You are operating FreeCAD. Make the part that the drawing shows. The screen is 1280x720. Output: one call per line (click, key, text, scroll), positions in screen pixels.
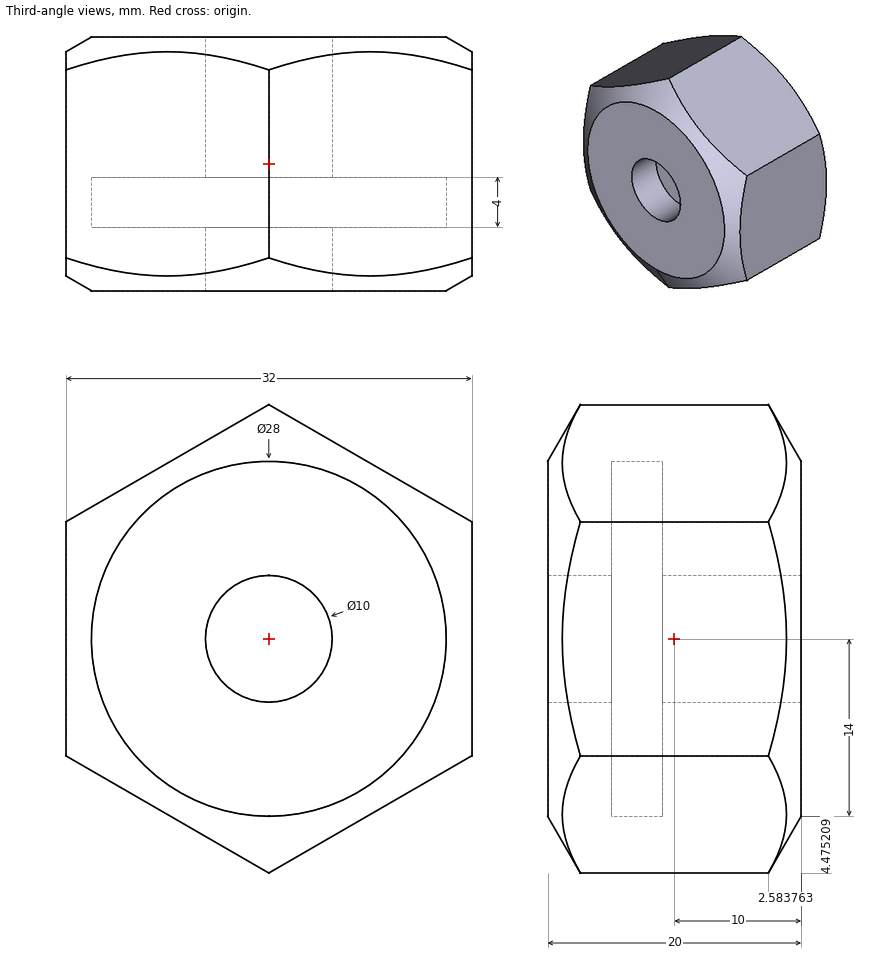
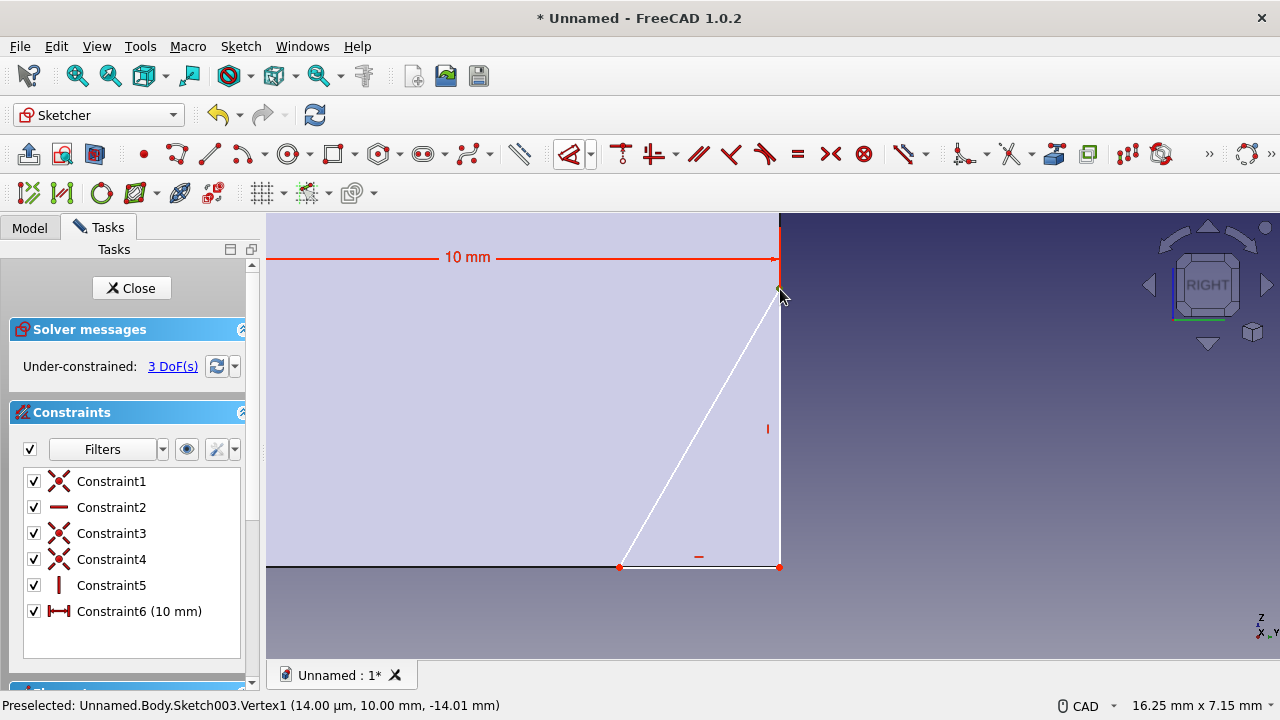
click(590, 154)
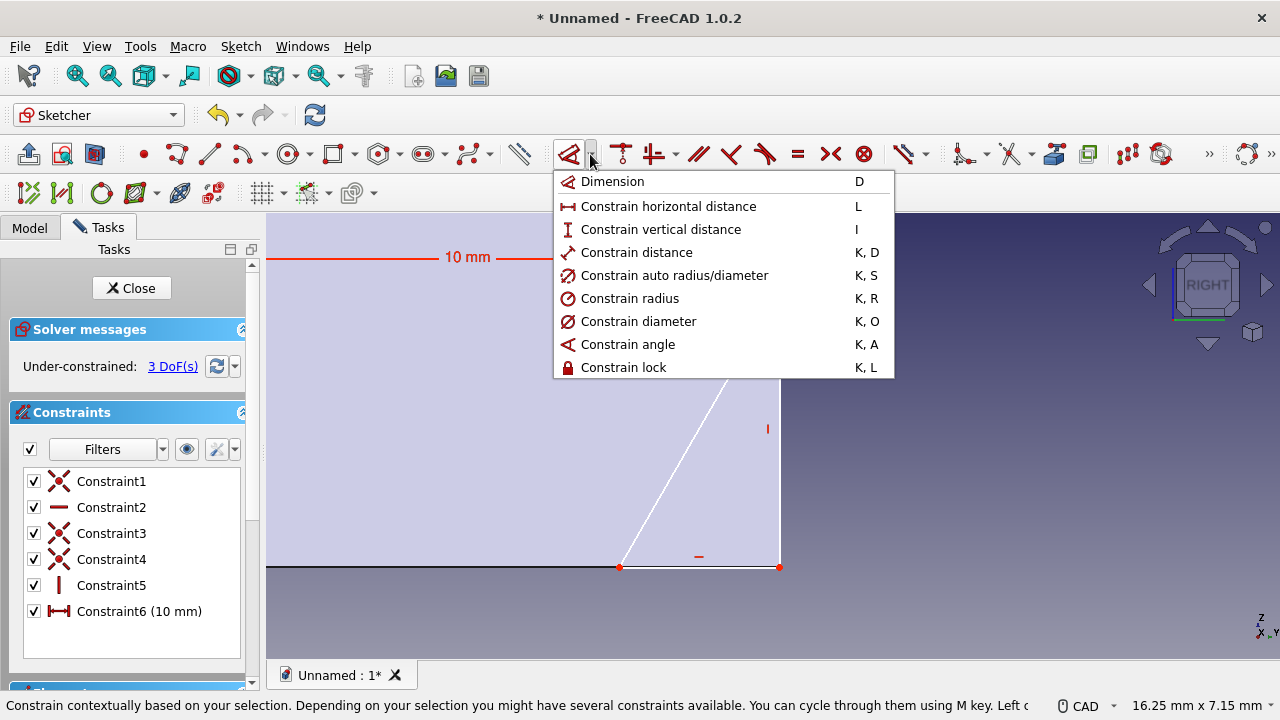
click(724, 230)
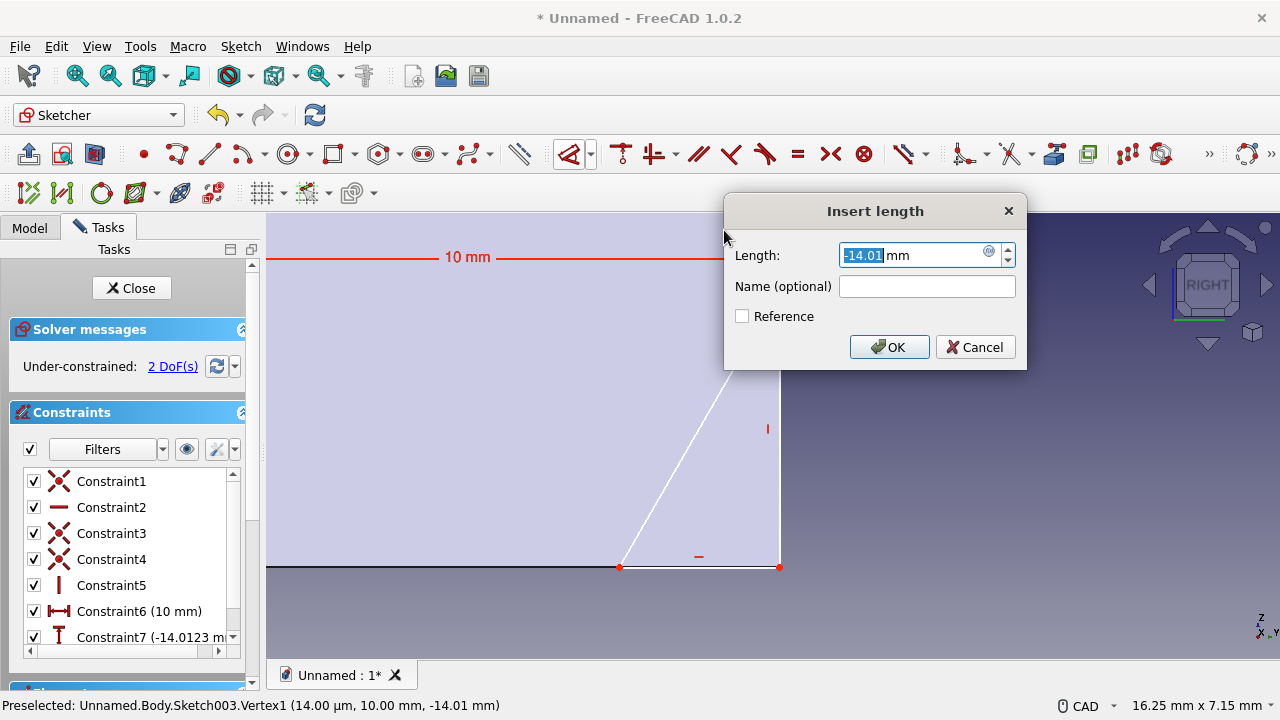
text(-14)
key(Return)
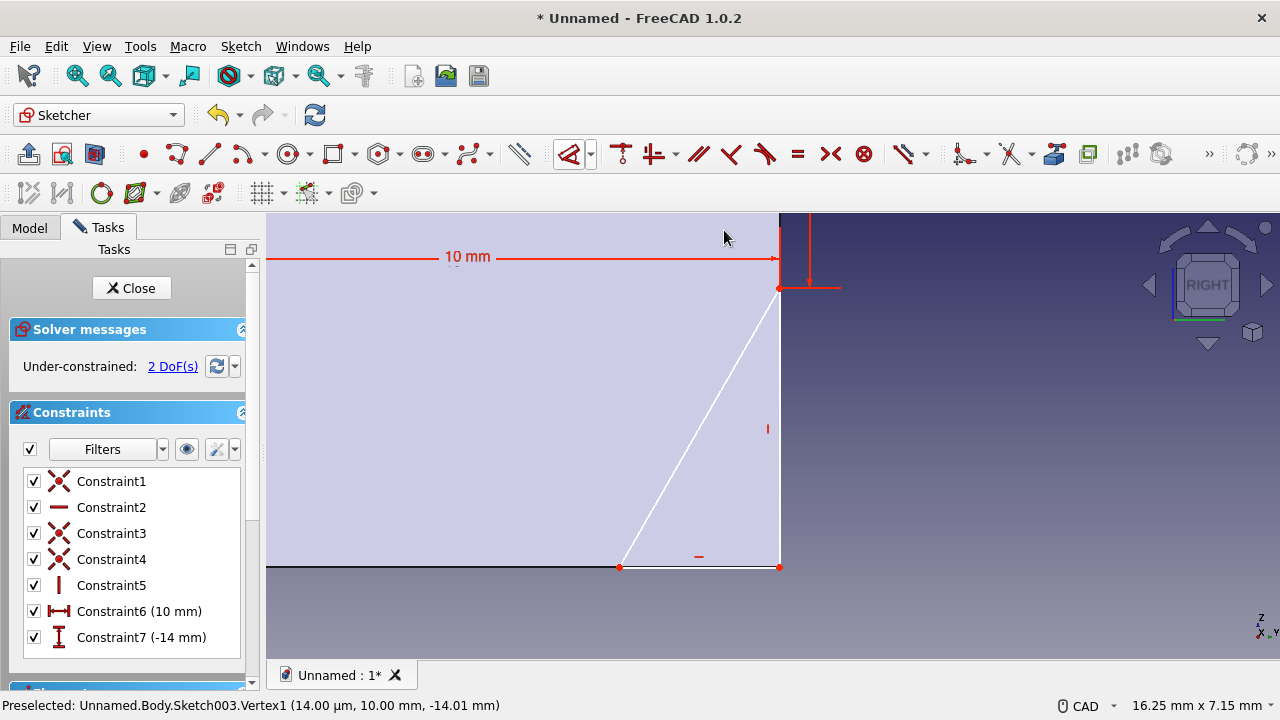
click(667, 568)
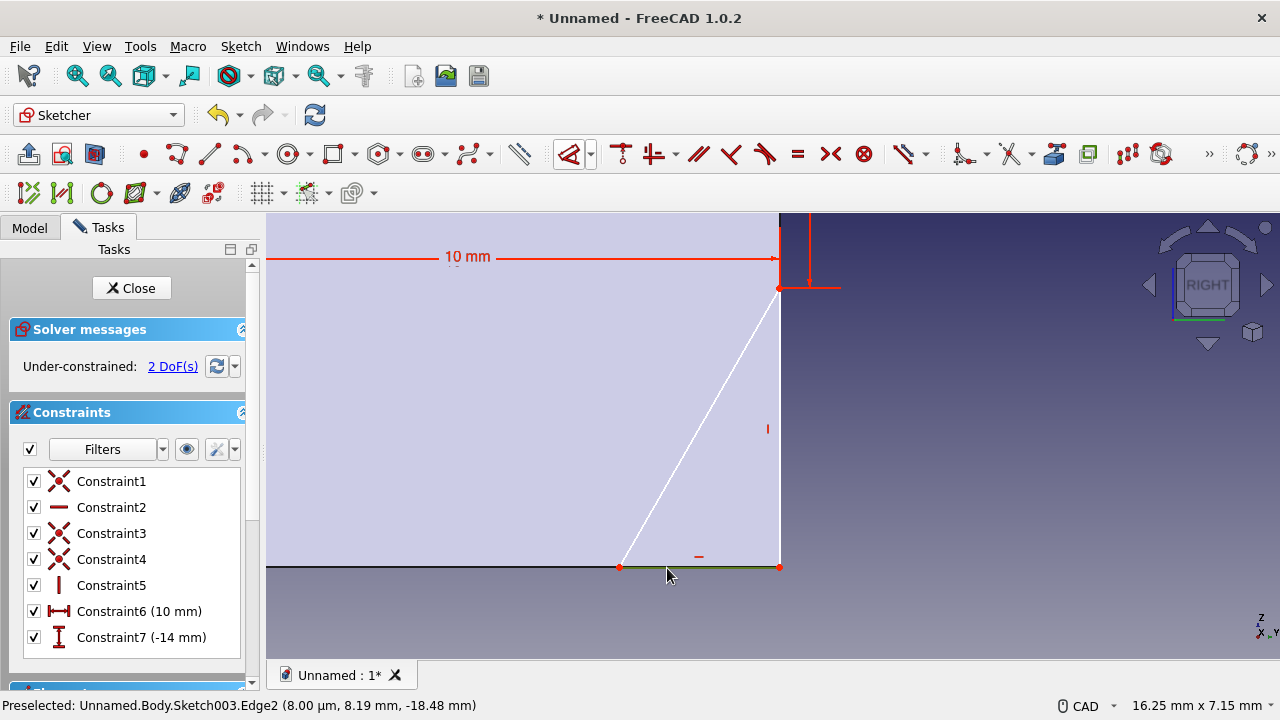
click(590, 154)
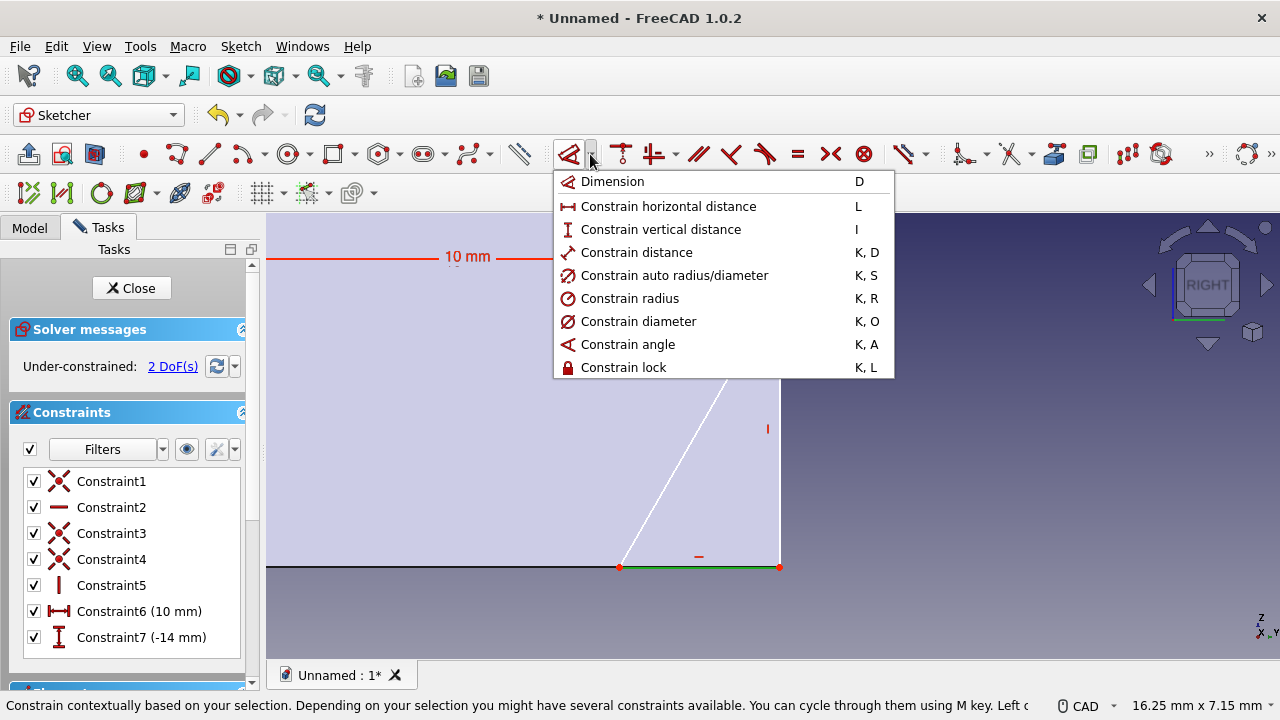
click(724, 206)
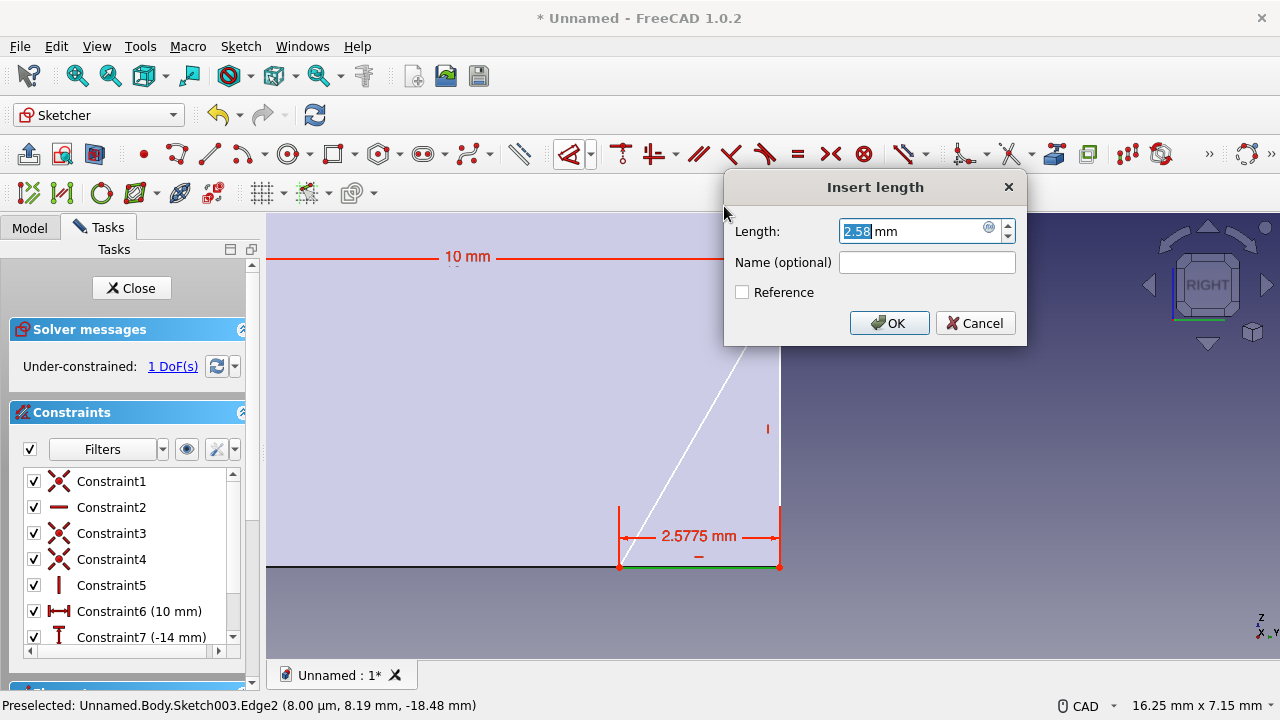
text(2.583763)
key(Return)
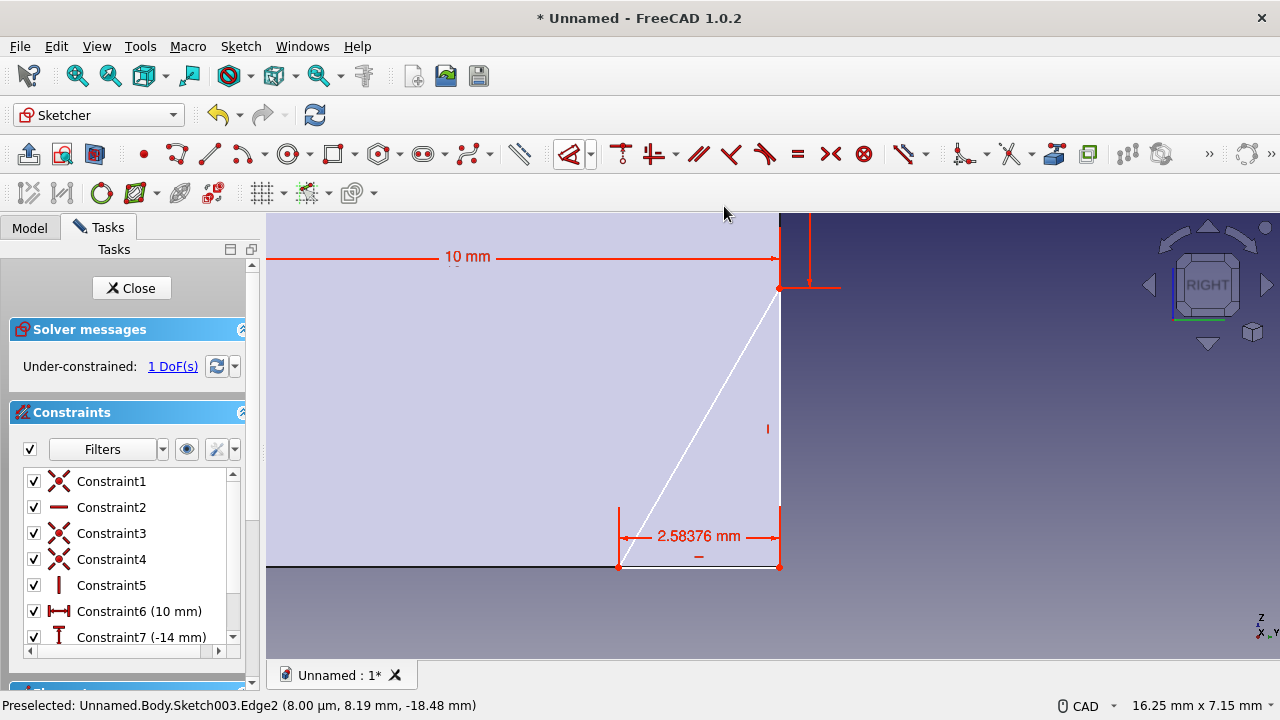
click(780, 484)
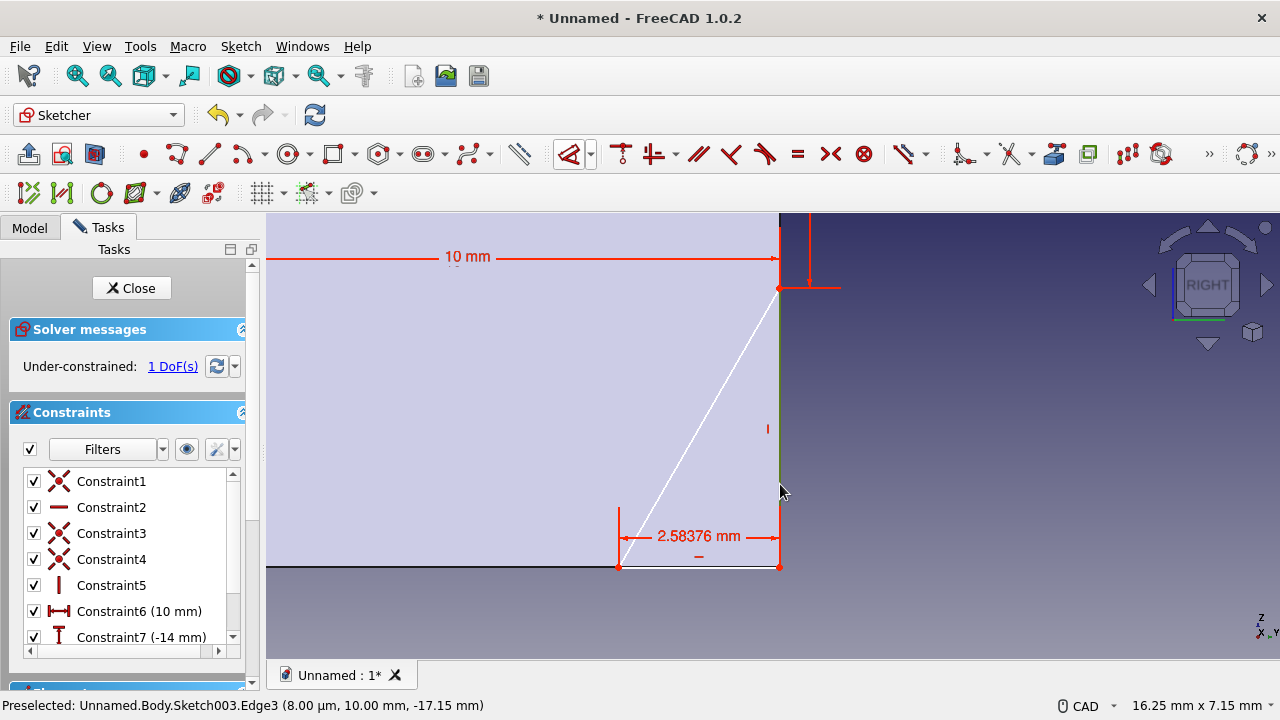
click(590, 154)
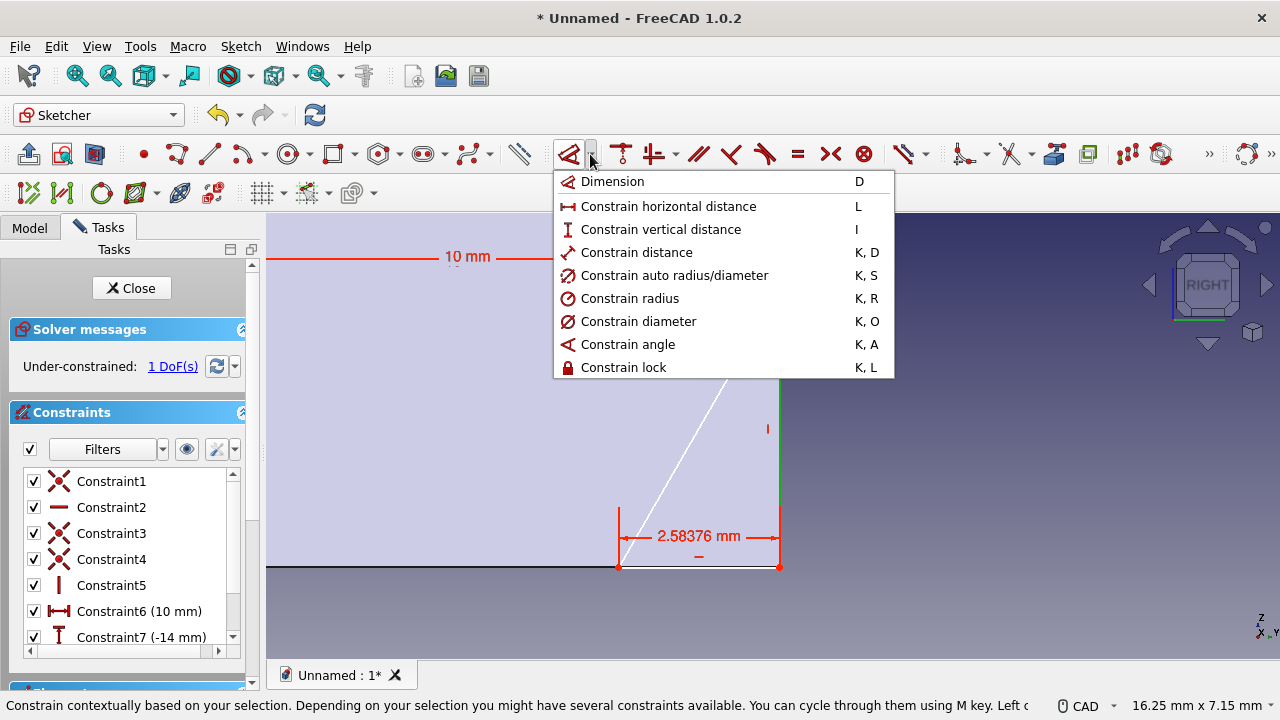
click(724, 230)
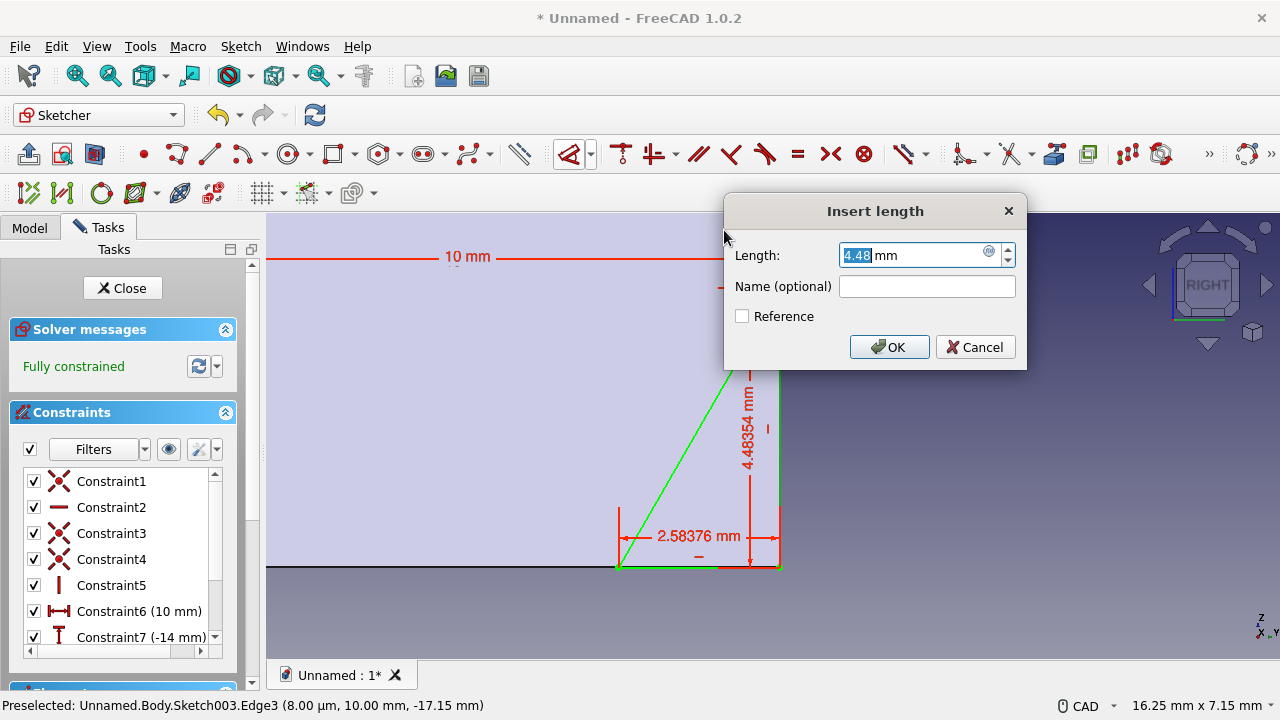
text(4.475209)
key(Return)